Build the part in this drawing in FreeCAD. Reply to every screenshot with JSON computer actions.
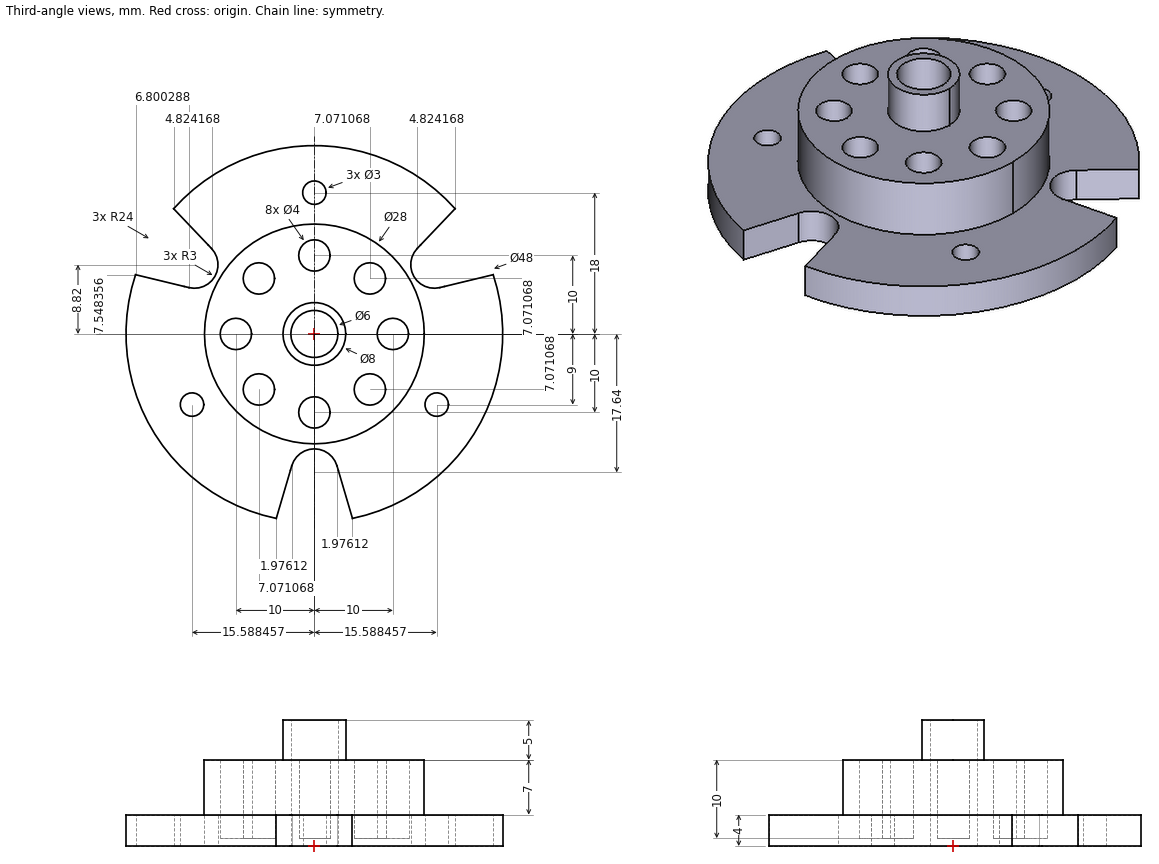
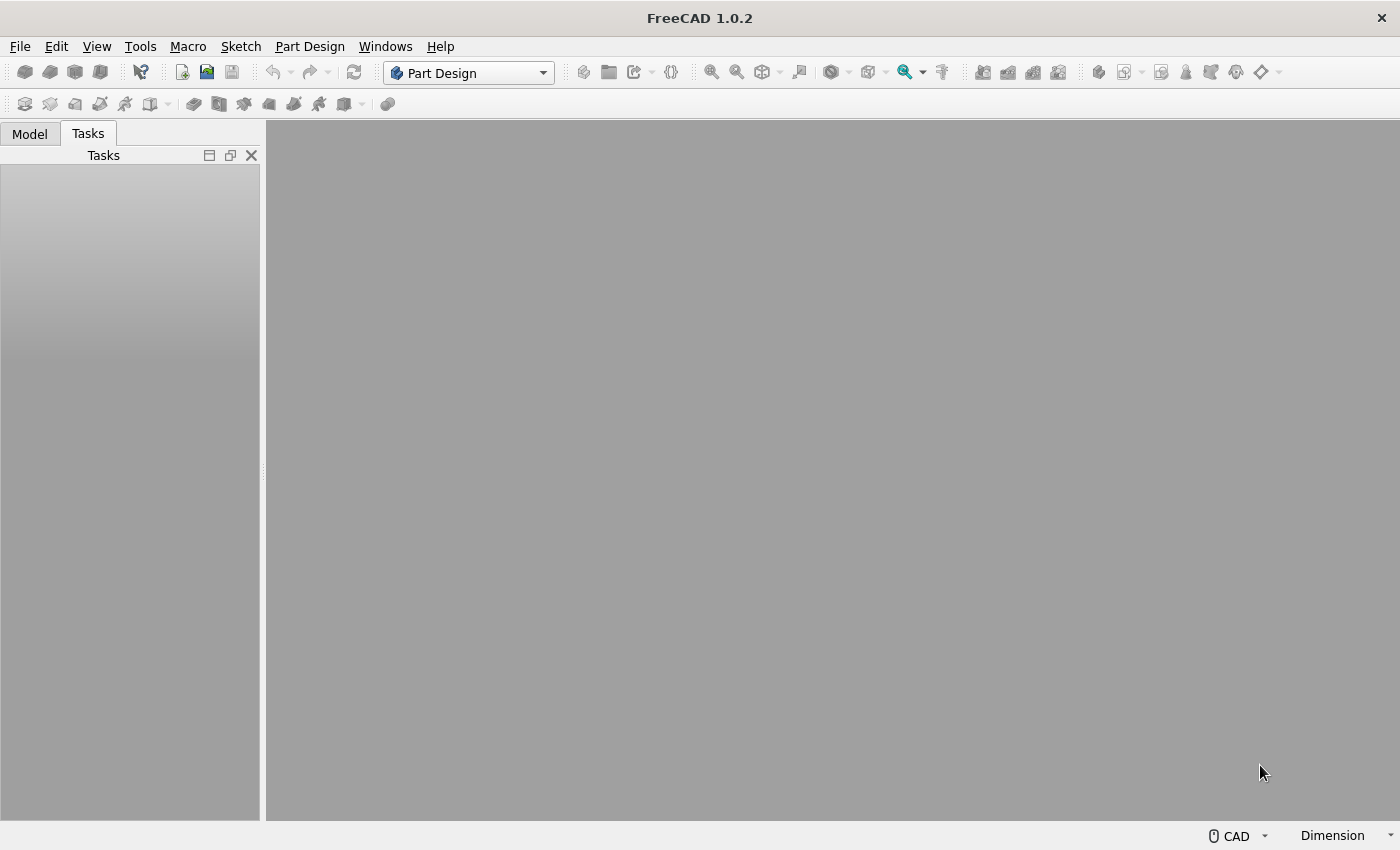
{"action": "key", "text": "ctrl+n"}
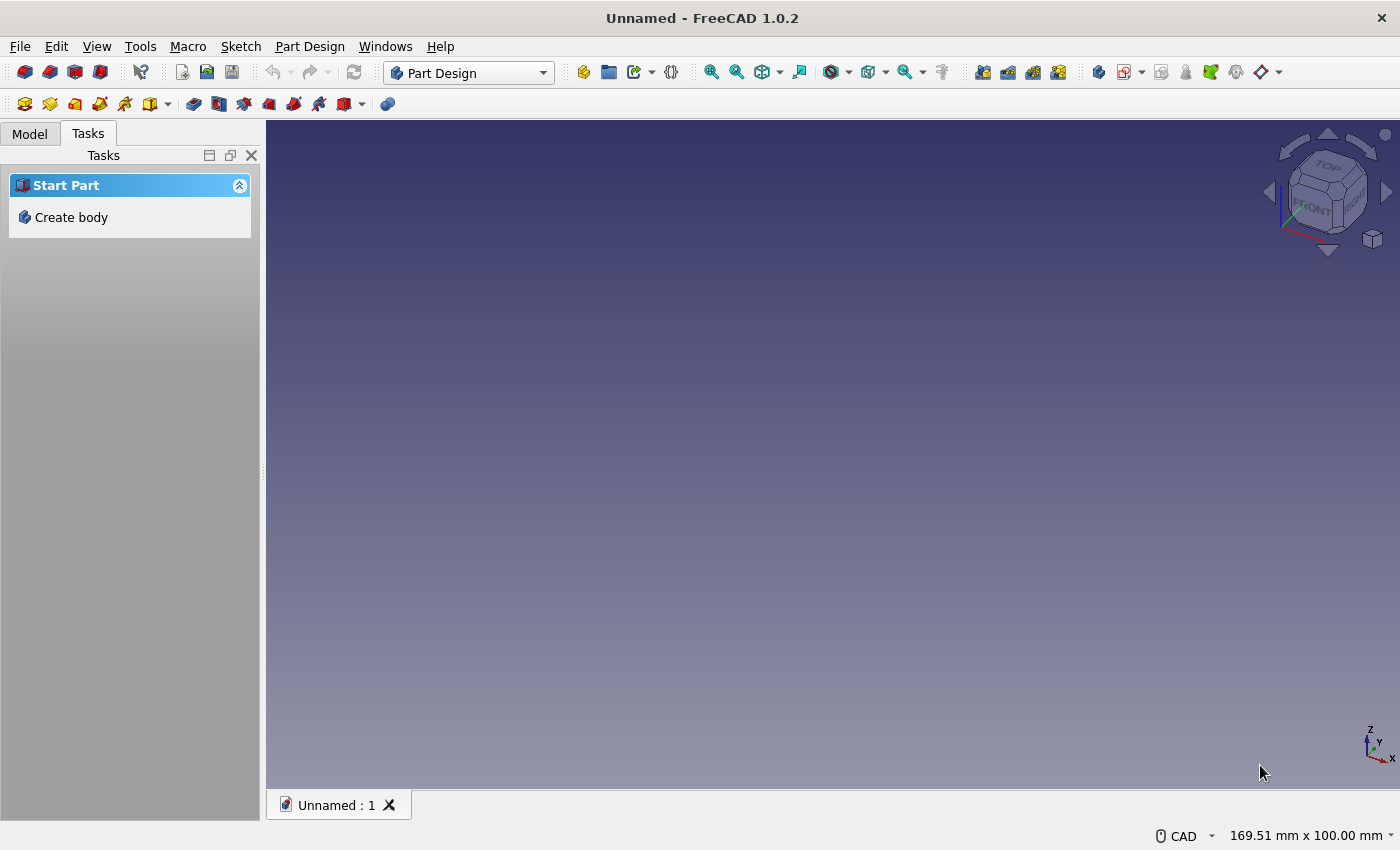
{"action": "left_click", "coordinate": [1124, 72]}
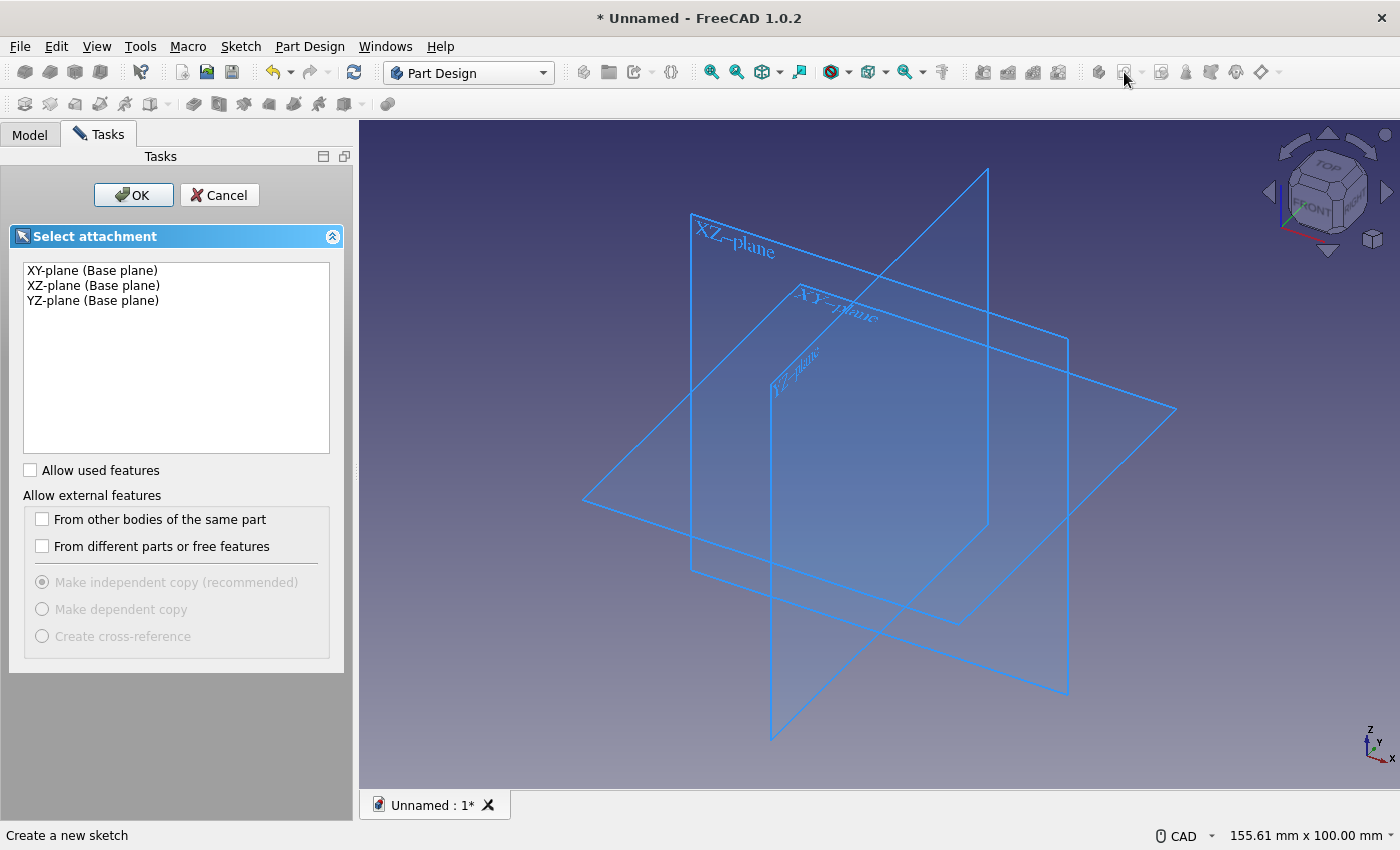
{"action": "left_click", "coordinate": [84, 270]}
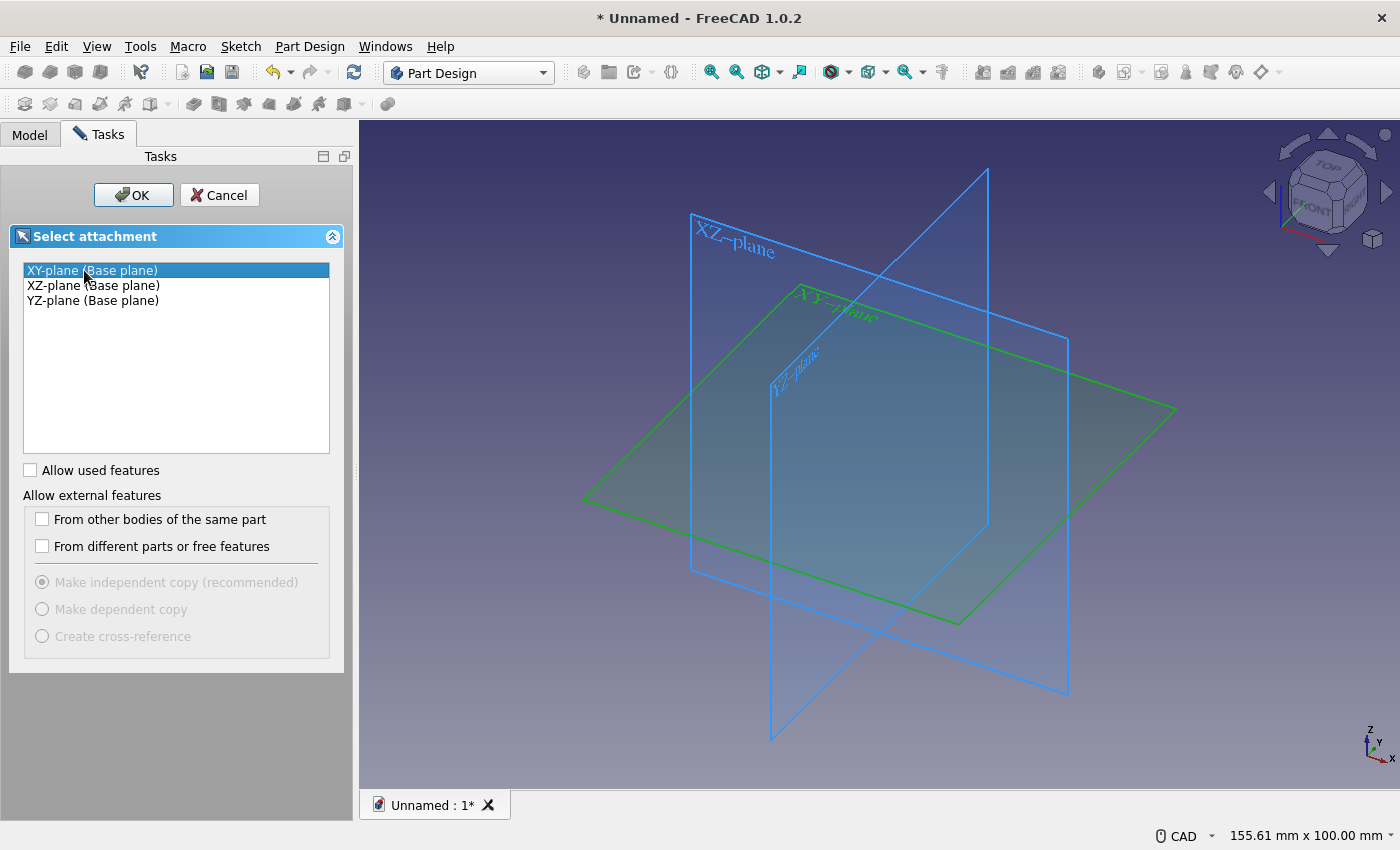
{"action": "left_click", "coordinate": [134, 195]}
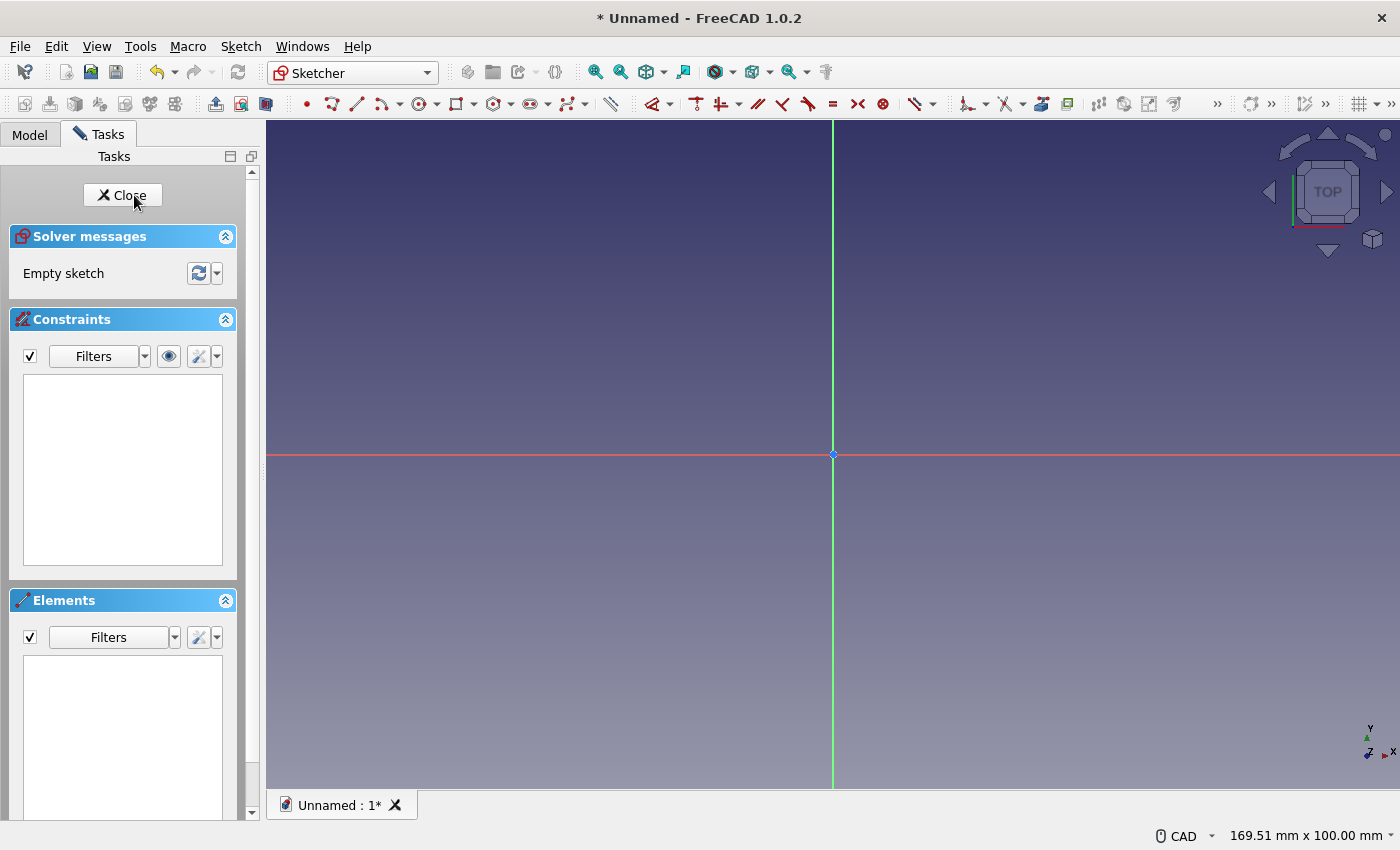
{"action": "key", "text": "g c"}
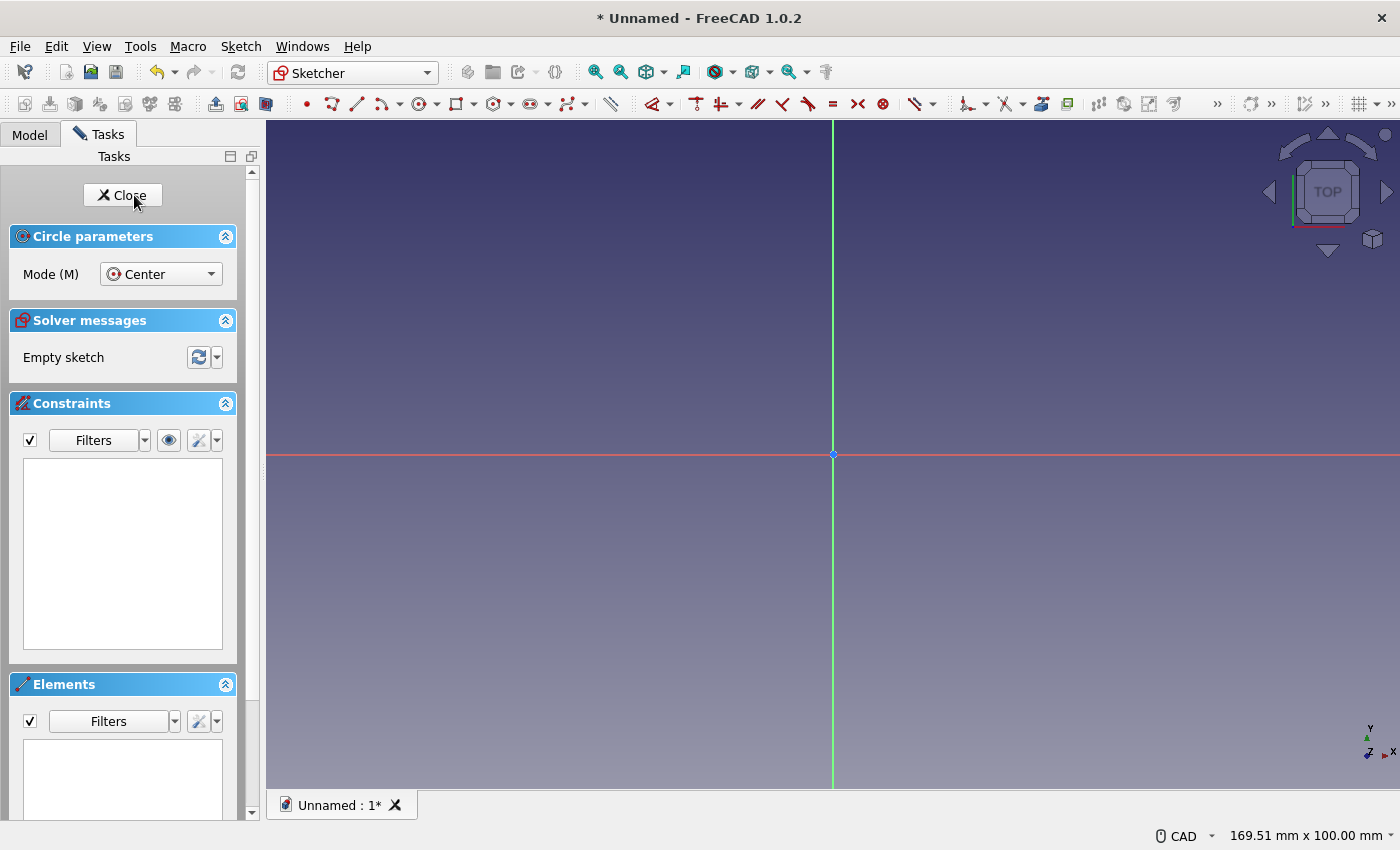
{"action": "left_click", "coordinate": [833, 454]}
{"action": "mouse_move", "coordinate": [947, 341]}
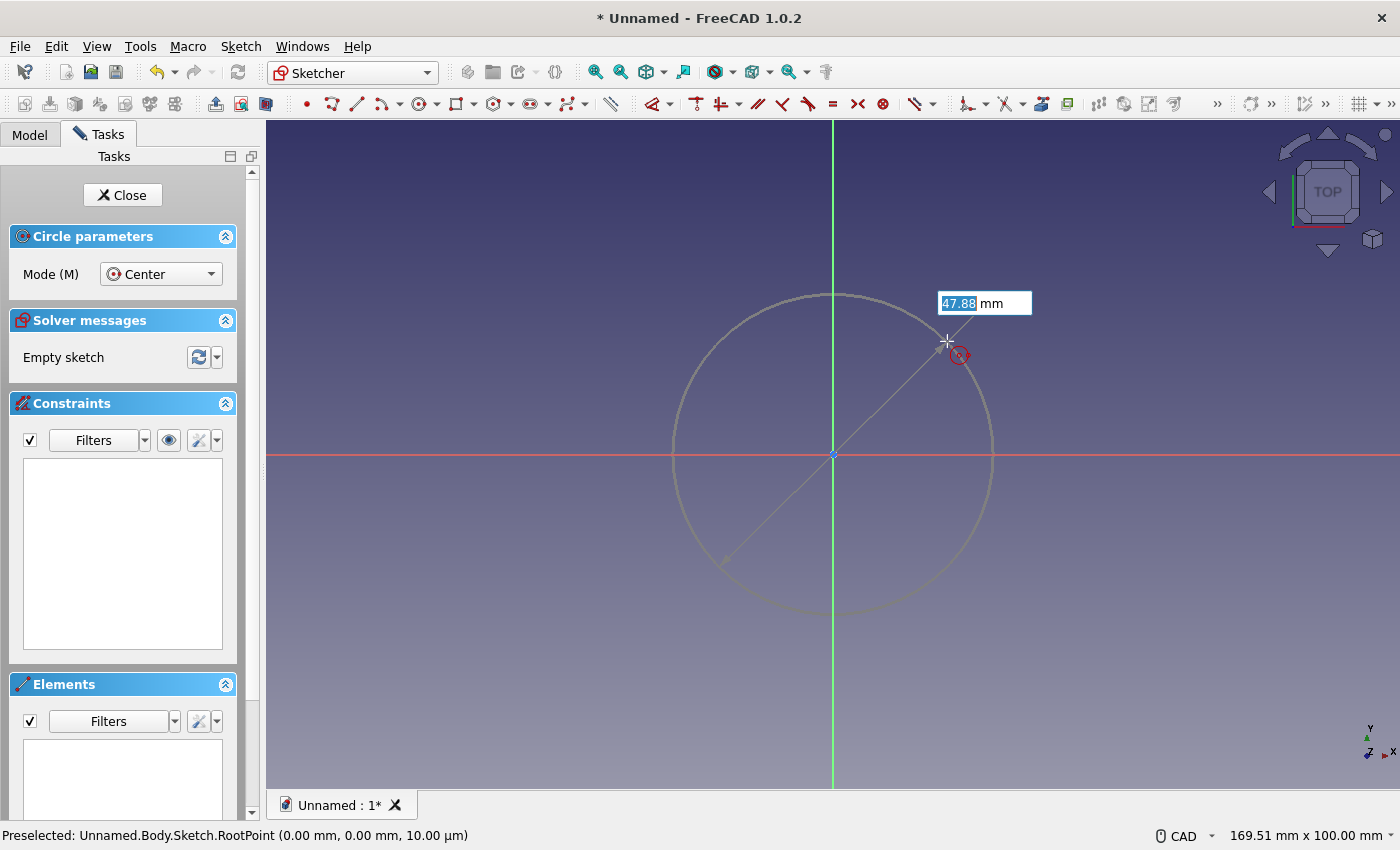
{"action": "type", "text": "48"}
{"action": "key", "text": "Return"}
{"action": "key", "text": "Escape"}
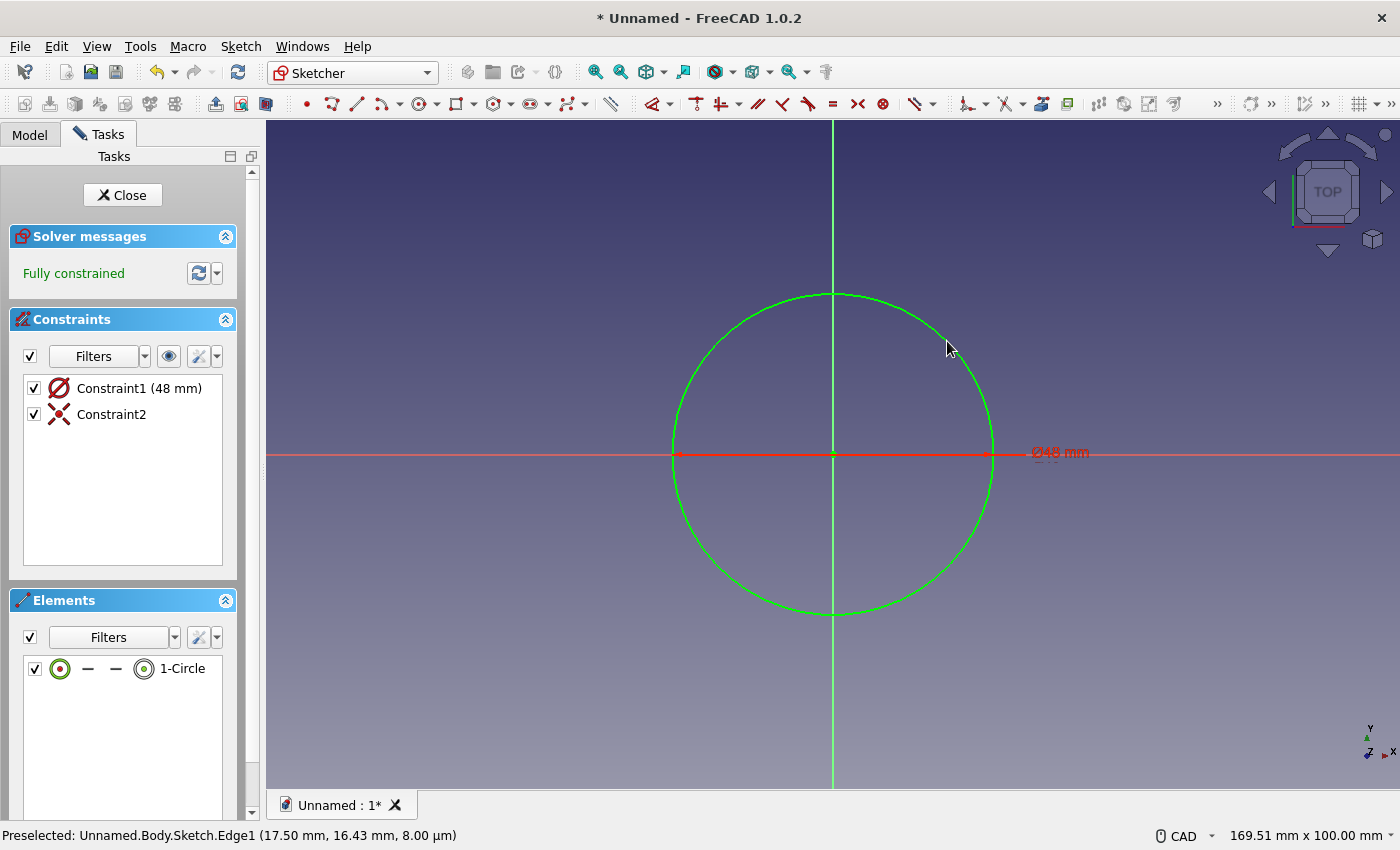
{"action": "left_click", "coordinate": [123, 195]}